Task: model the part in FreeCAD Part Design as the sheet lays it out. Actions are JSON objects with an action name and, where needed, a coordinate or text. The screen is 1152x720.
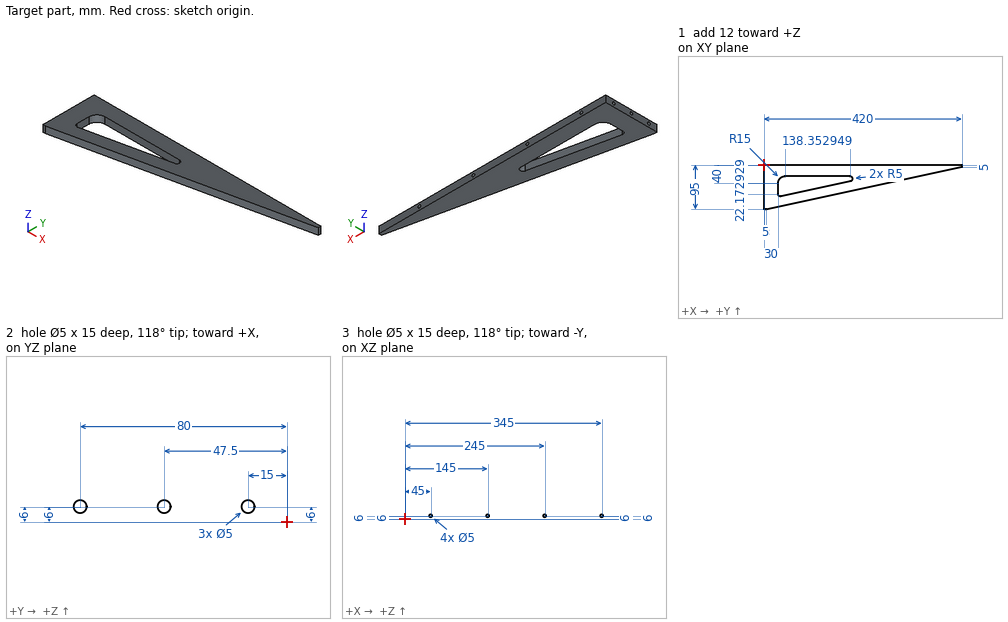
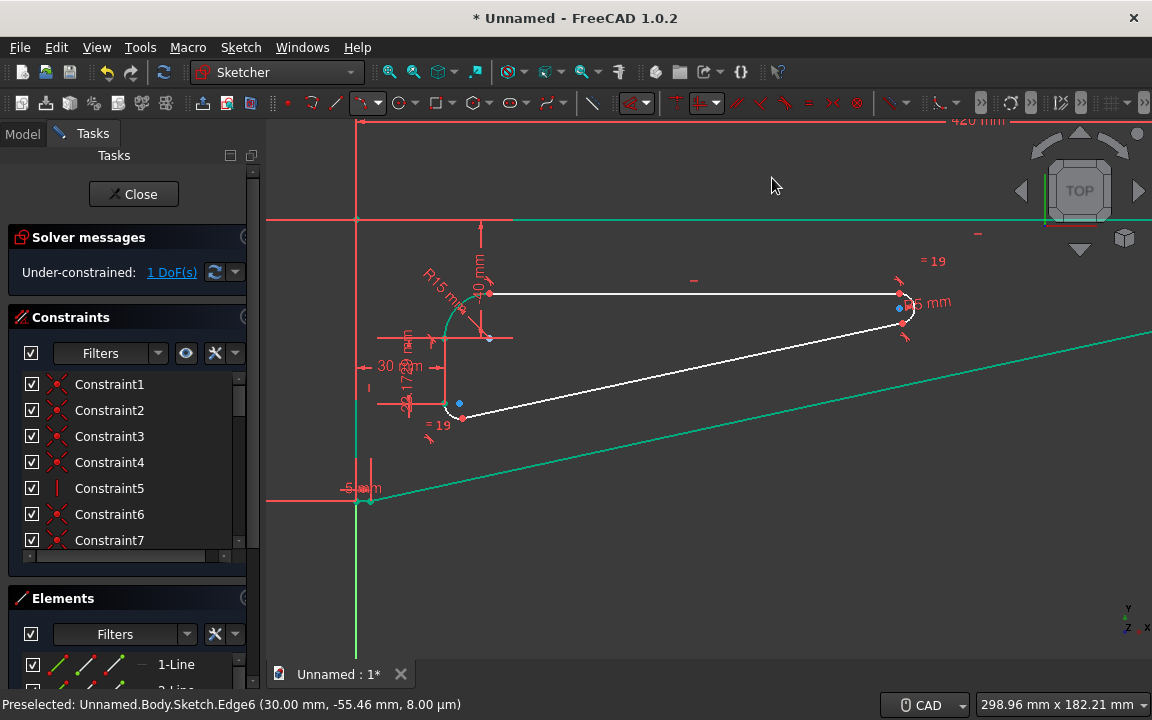
{"action": "left_click", "coordinate": [612, 294]}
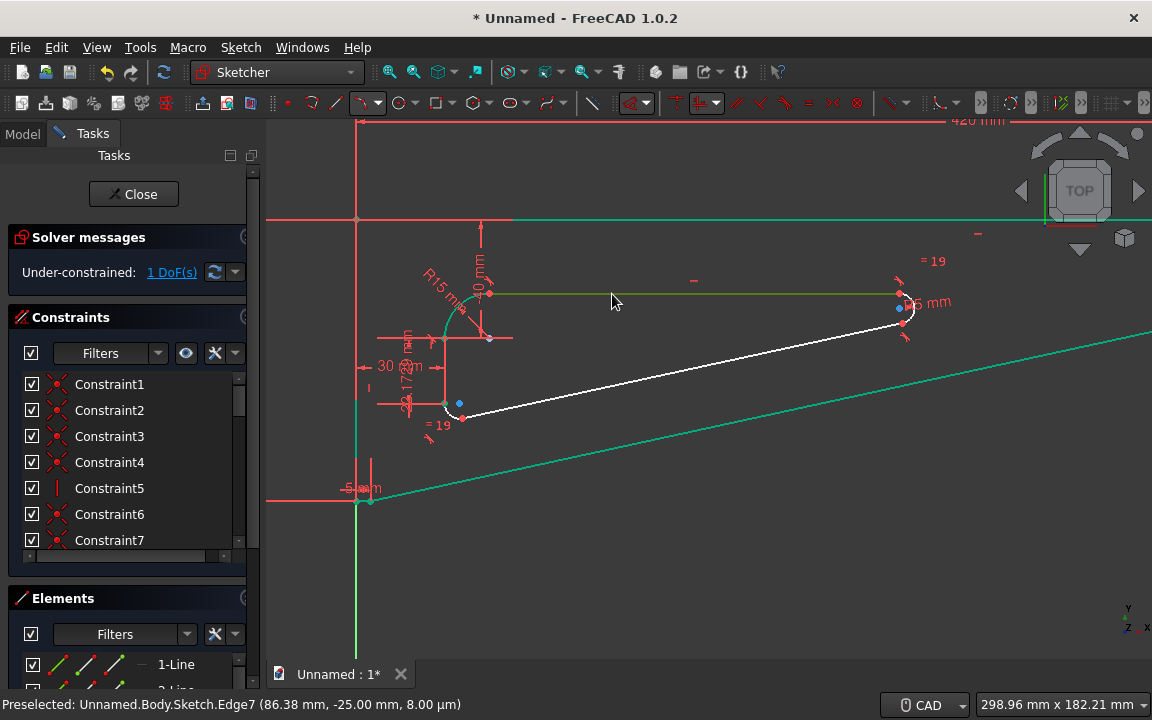
{"action": "left_click", "coordinate": [648, 104]}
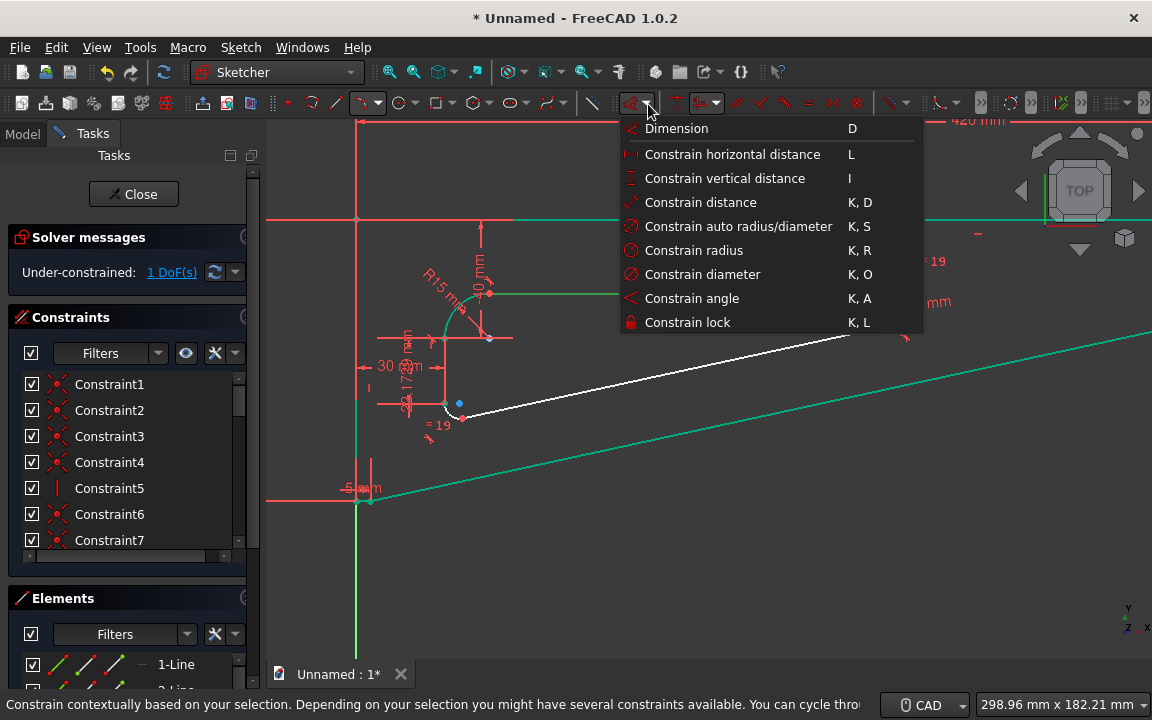
{"action": "left_click", "coordinate": [772, 154]}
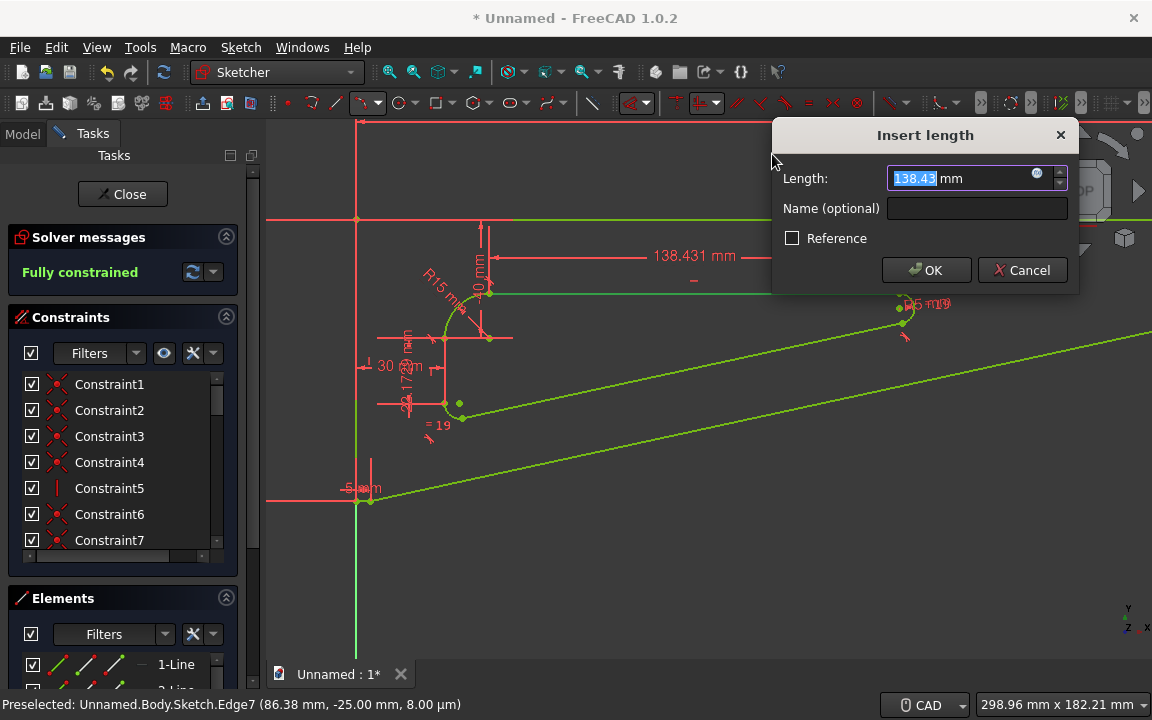
{"action": "type", "text": "138.352949"}
{"action": "key", "text": "Return"}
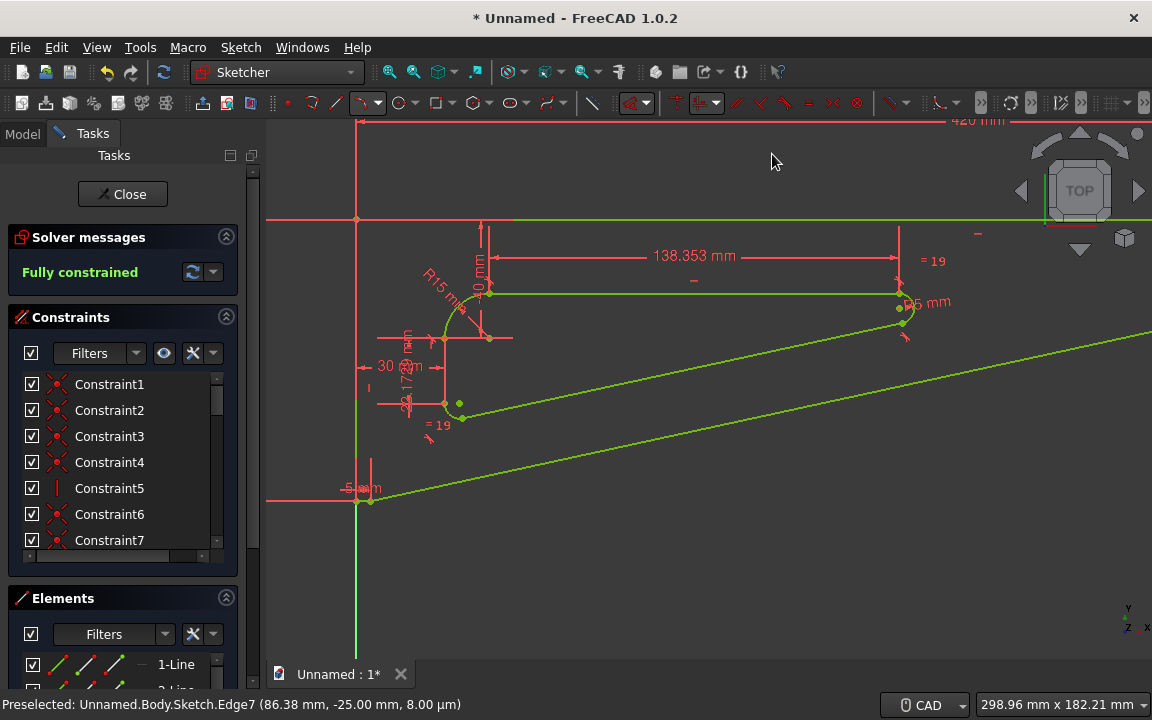
{"action": "left_click", "coordinate": [123, 194]}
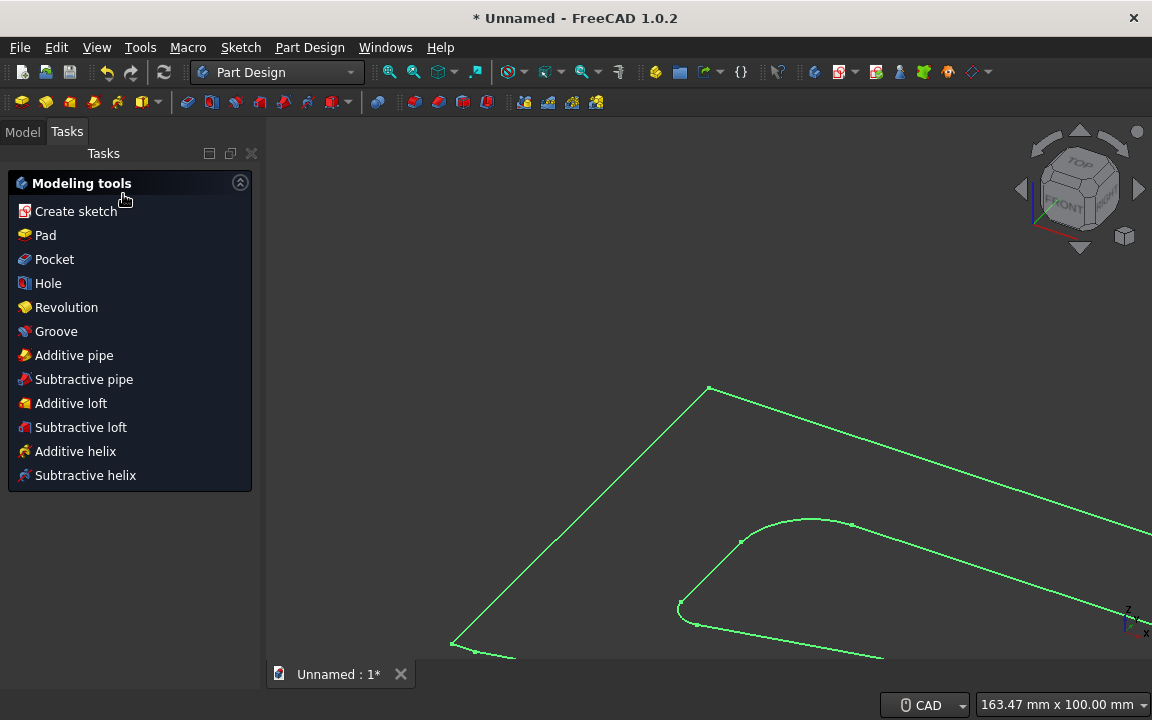
{"action": "left_click", "coordinate": [22, 102]}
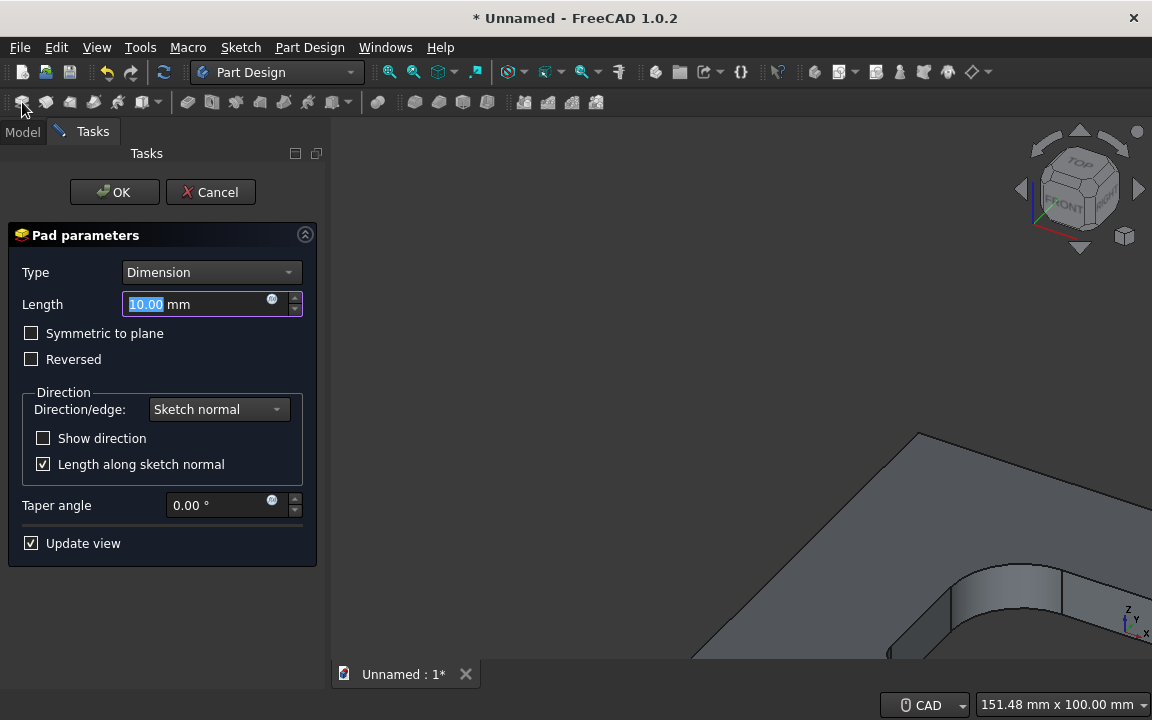
{"action": "type", "text": "12"}
{"action": "key", "text": "Tab"}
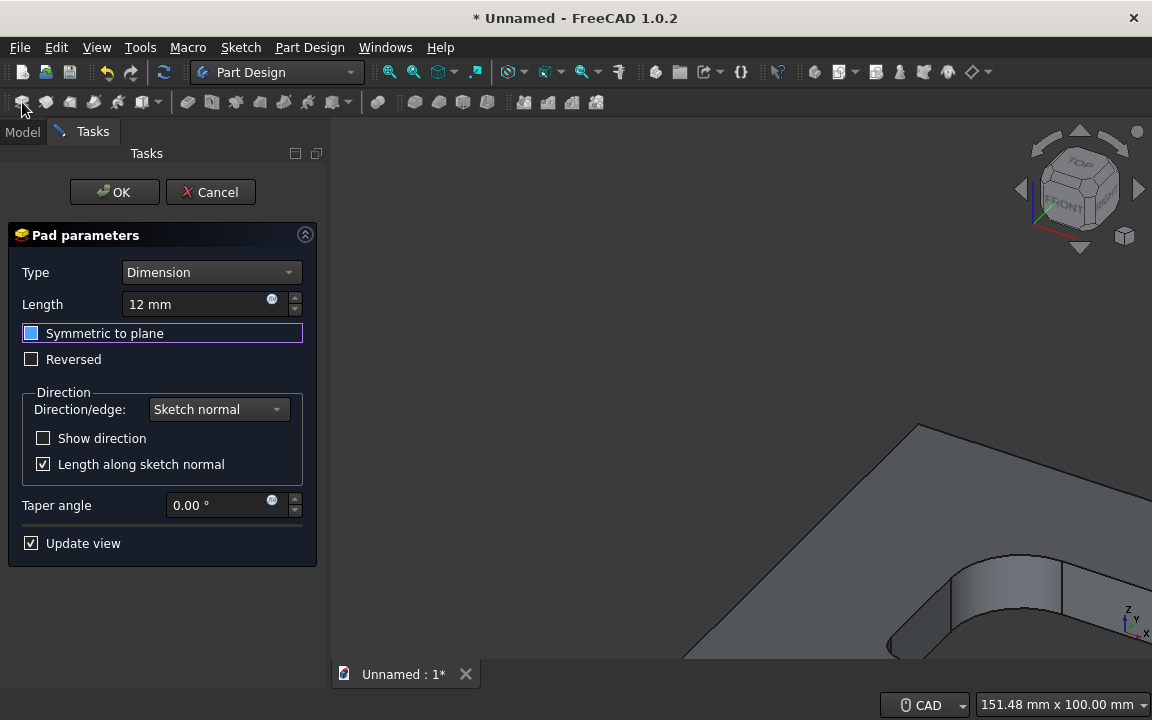
{"action": "left_click", "coordinate": [115, 192]}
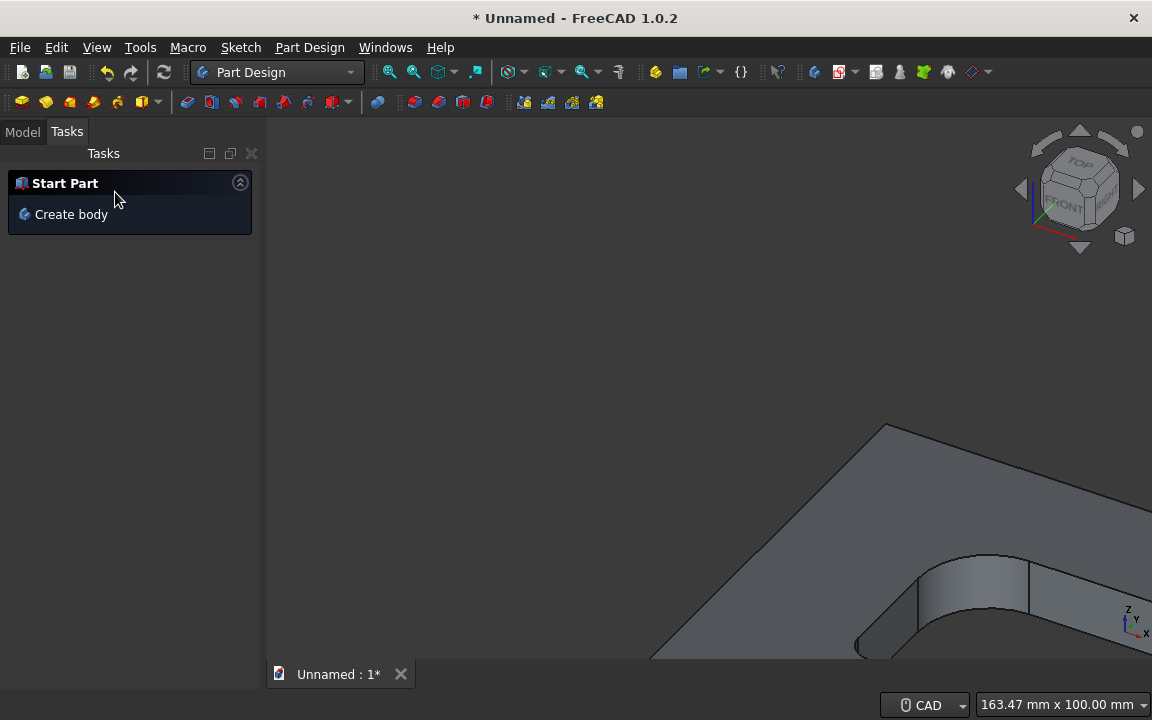
{"action": "left_click", "coordinate": [390, 72]}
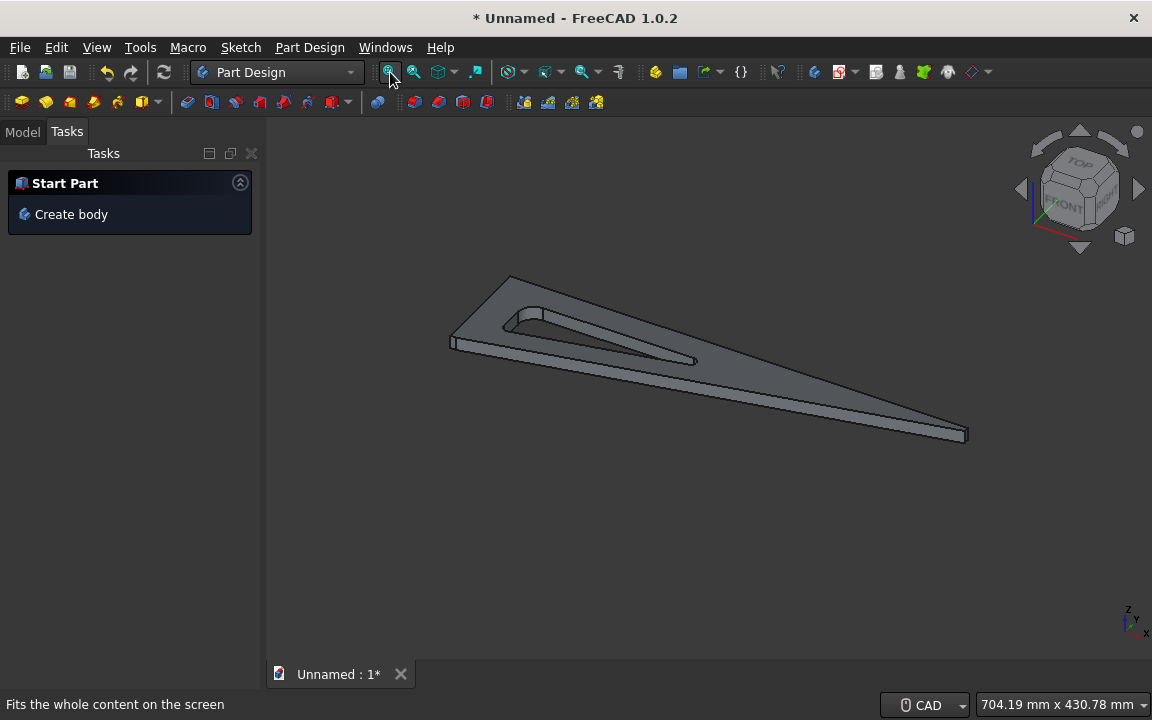
{"action": "left_click", "coordinate": [840, 72]}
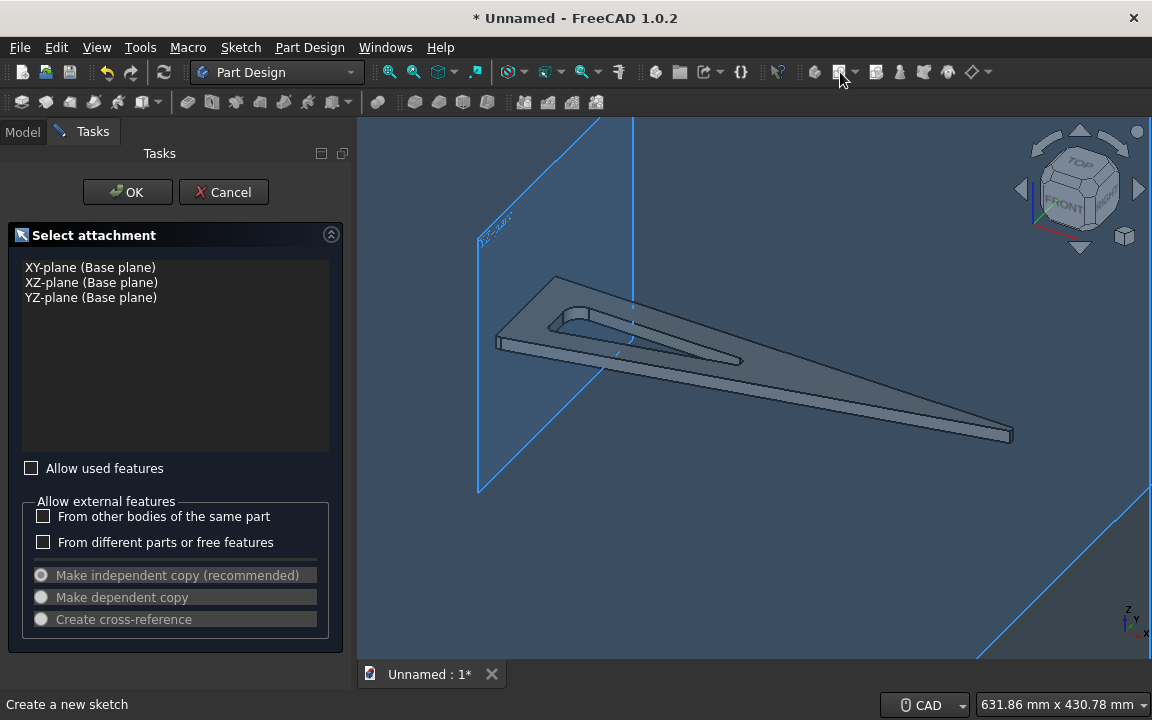
{"action": "left_click", "coordinate": [82, 298]}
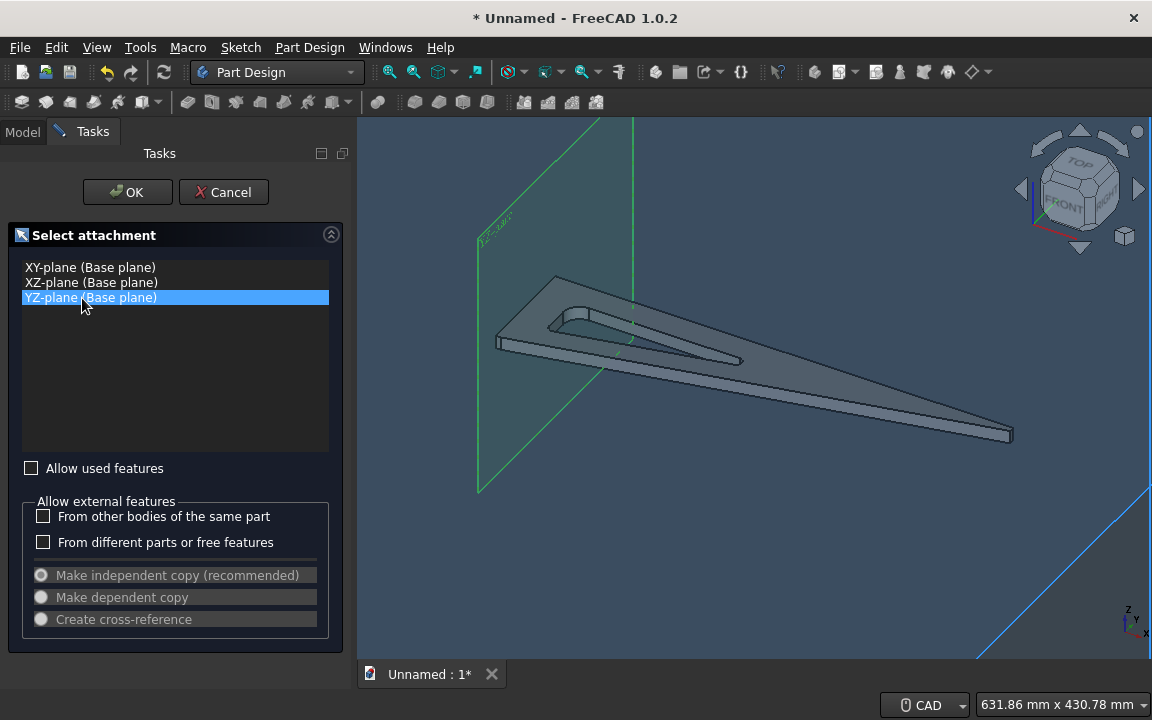
{"action": "left_click", "coordinate": [128, 192]}